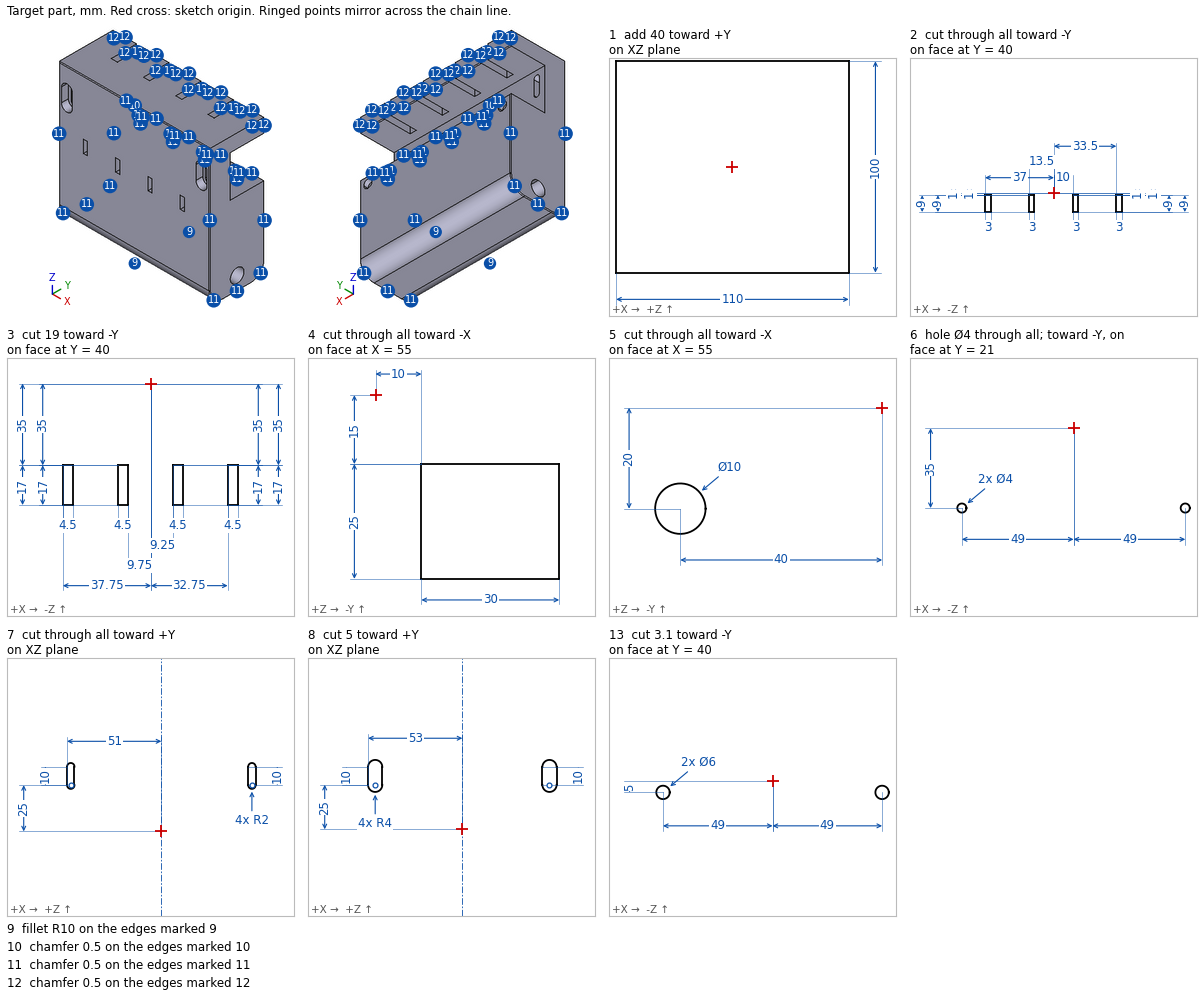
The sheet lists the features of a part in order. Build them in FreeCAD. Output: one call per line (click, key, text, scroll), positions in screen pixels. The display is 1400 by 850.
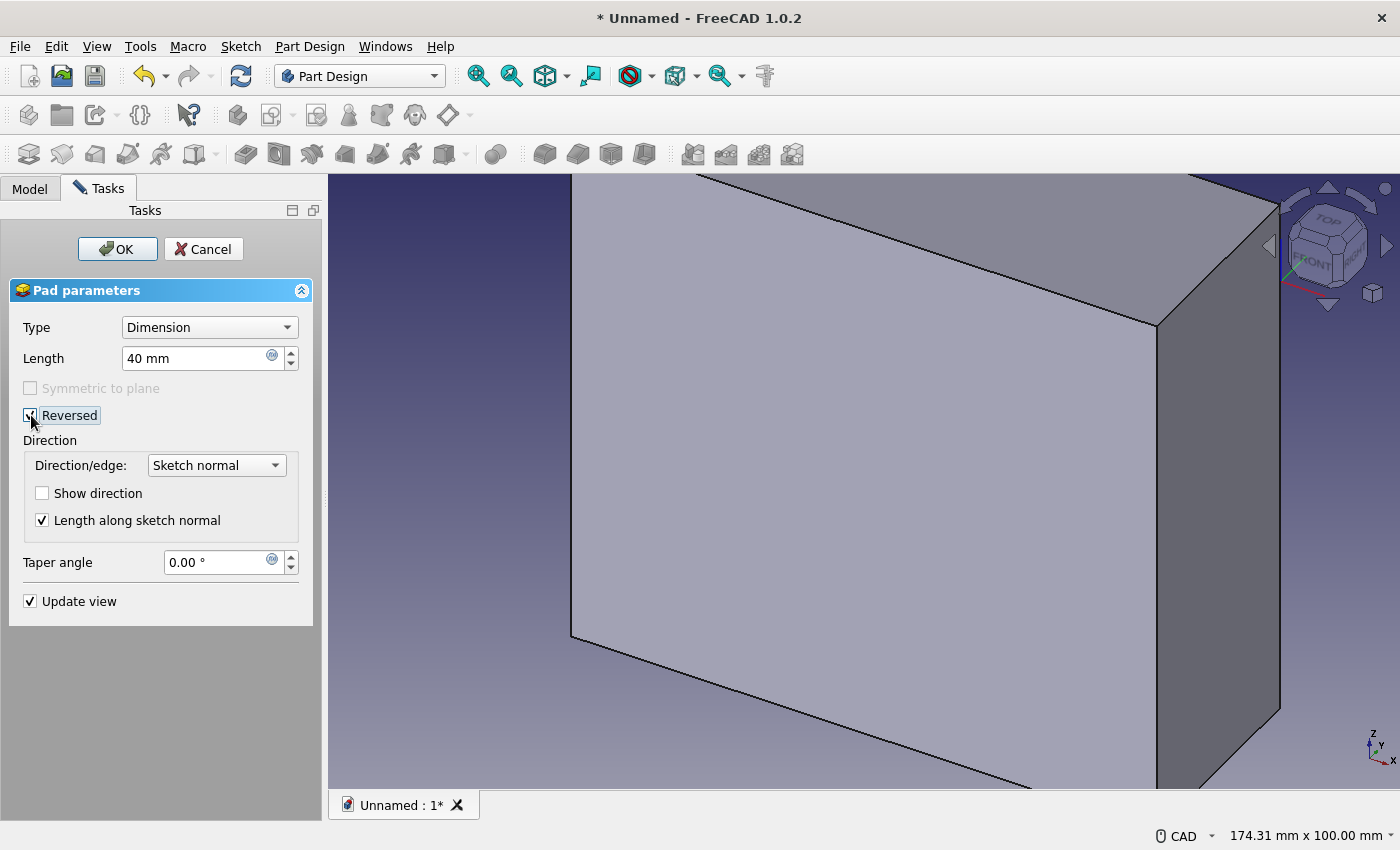
click(118, 249)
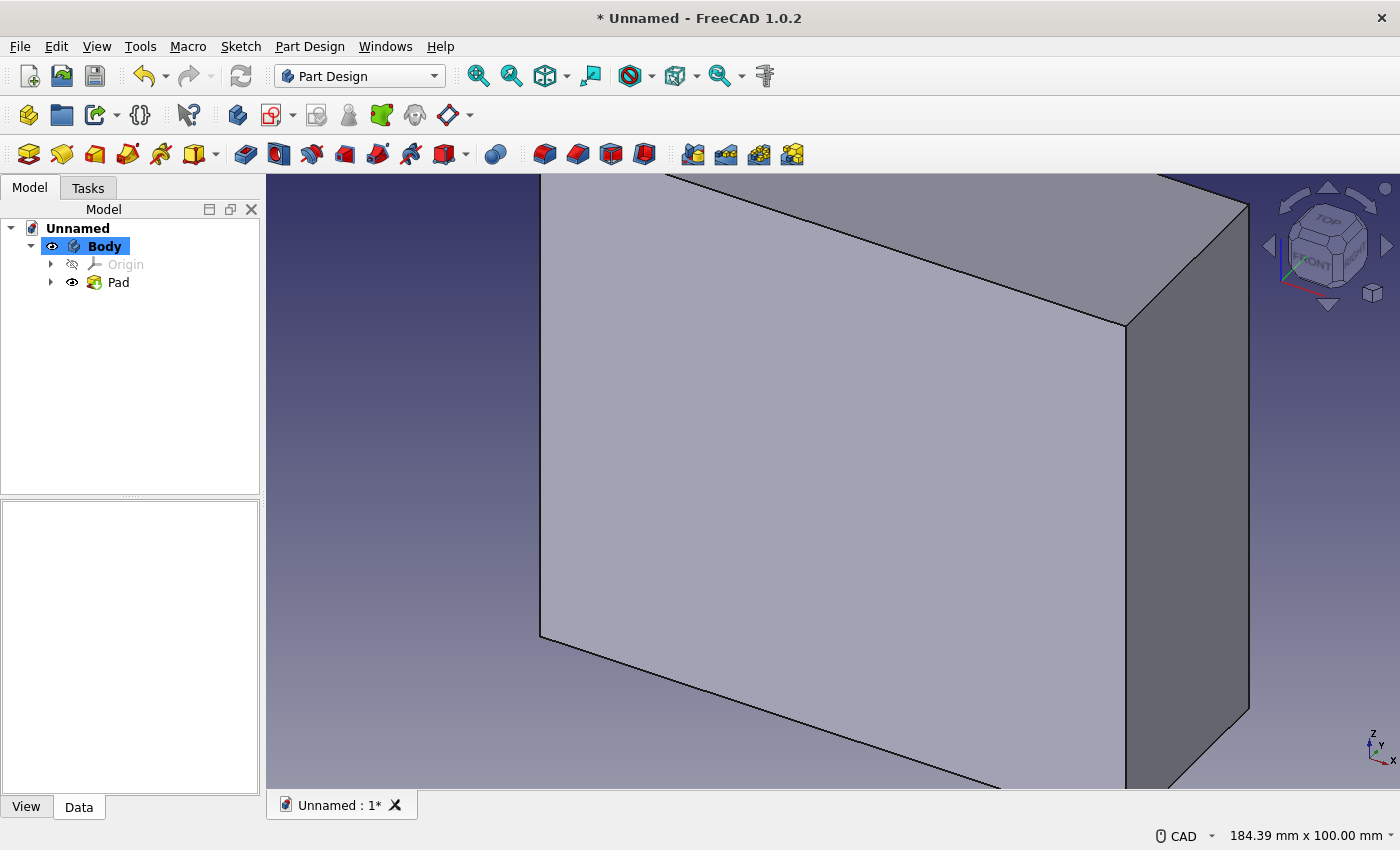
click(479, 76)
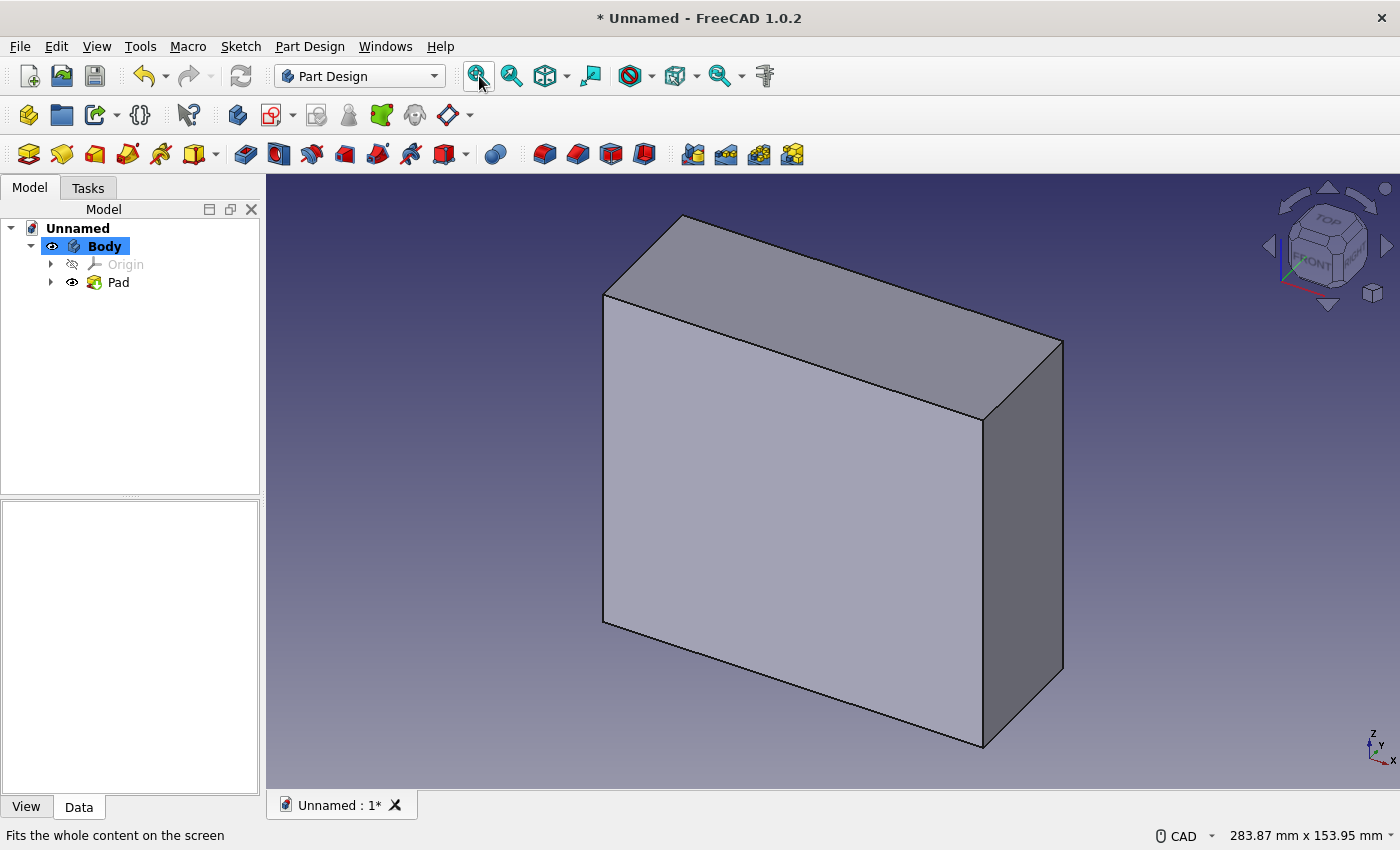
key(4)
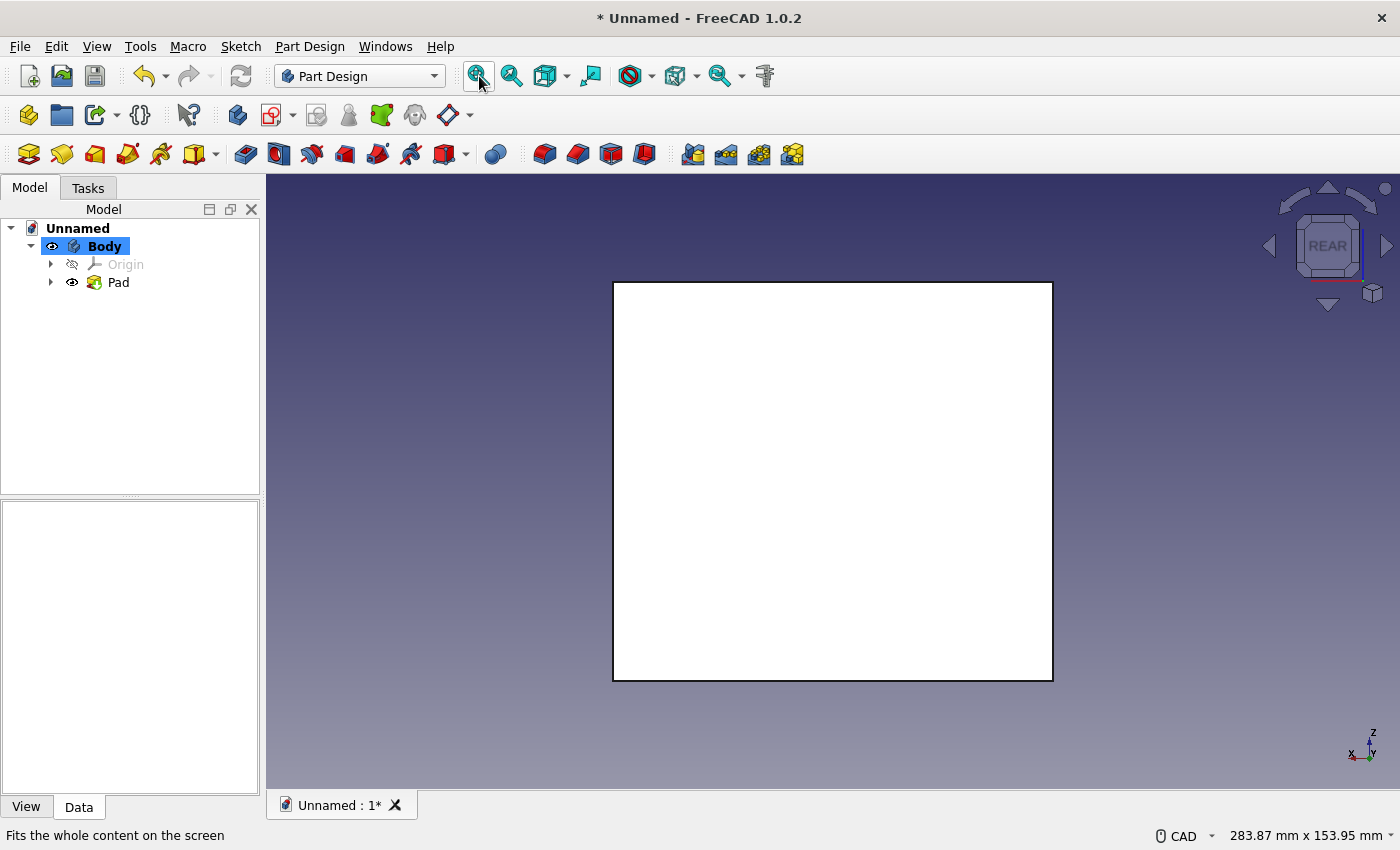
click(833, 481)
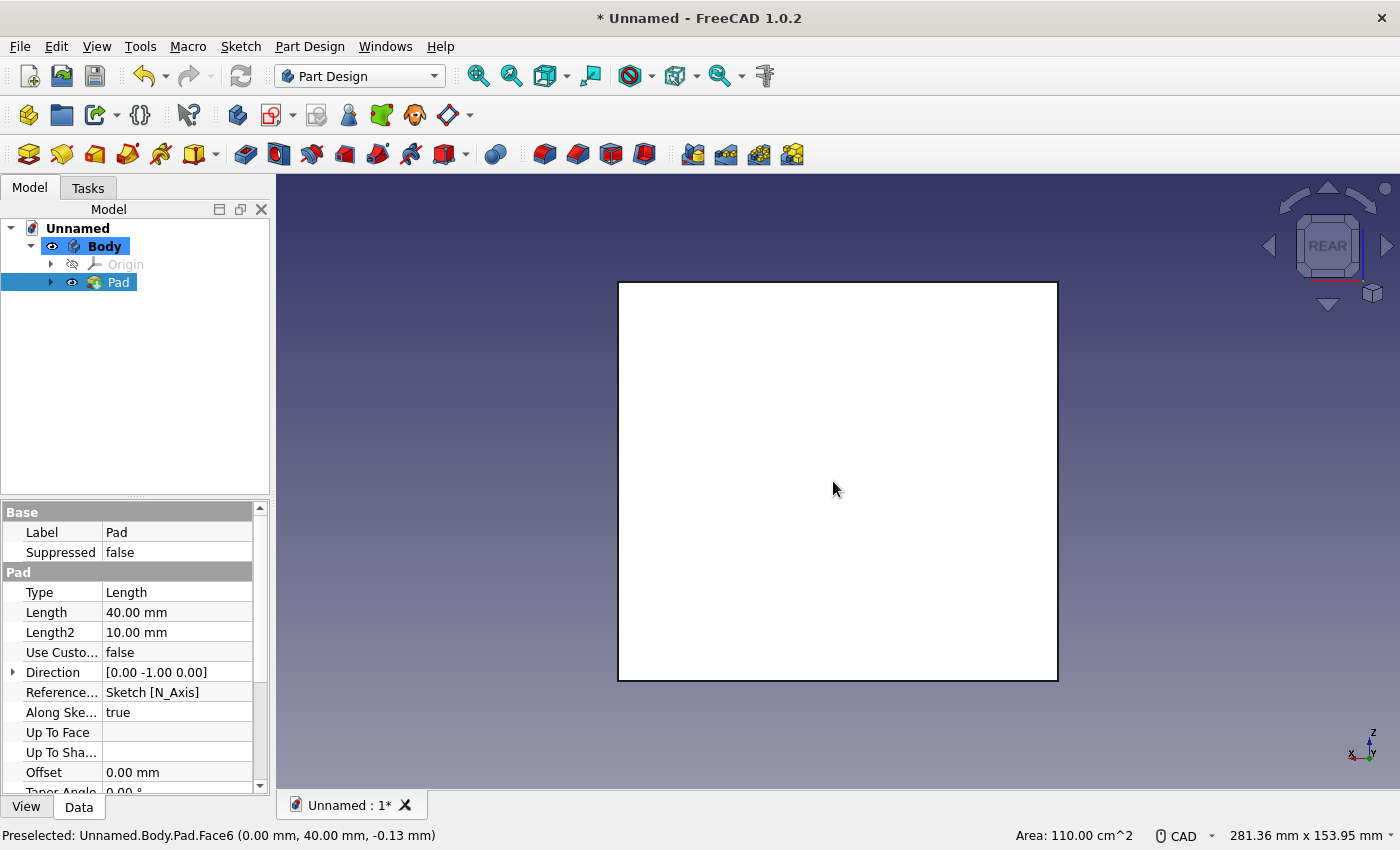
click(270, 116)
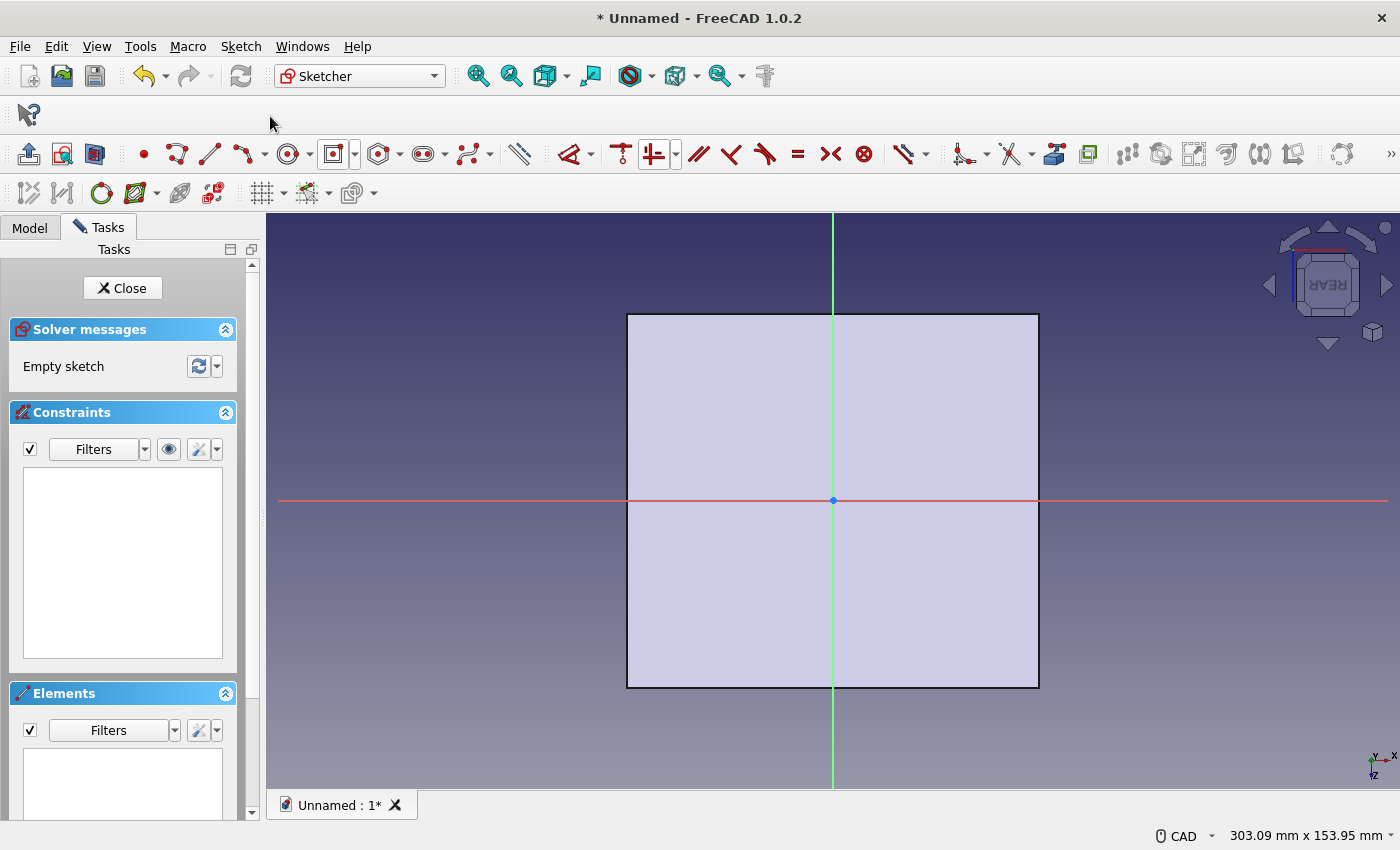
scroll(887, 535, up, 4)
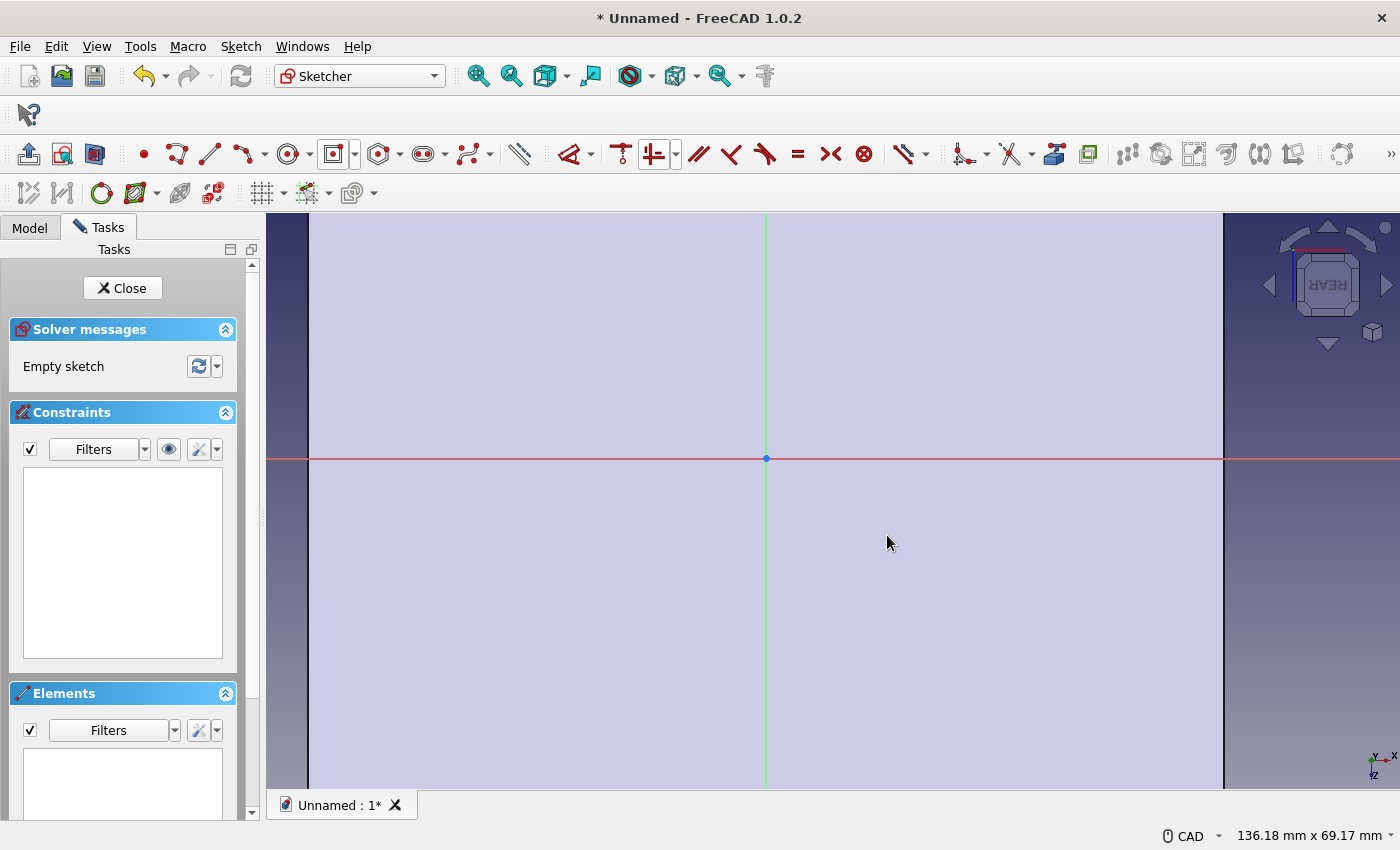
key(g)
key(r)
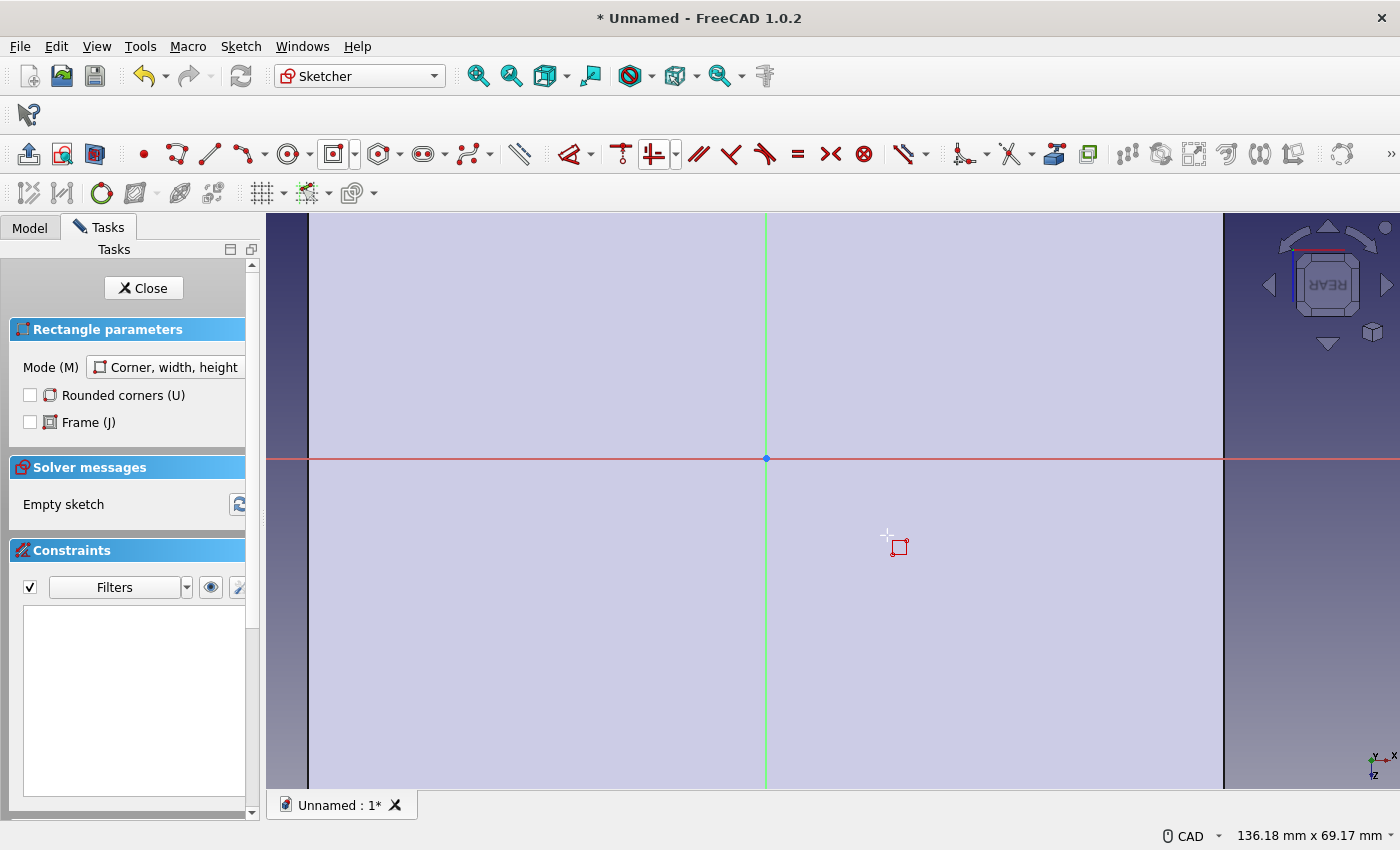
scroll(458, 467, up, 4)